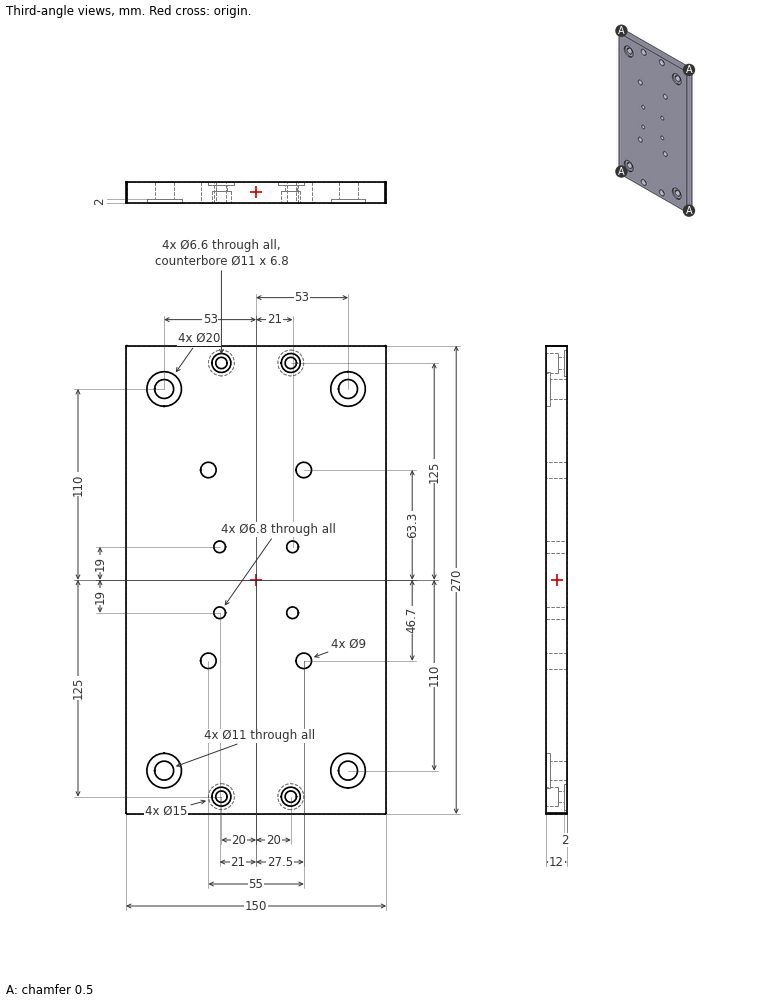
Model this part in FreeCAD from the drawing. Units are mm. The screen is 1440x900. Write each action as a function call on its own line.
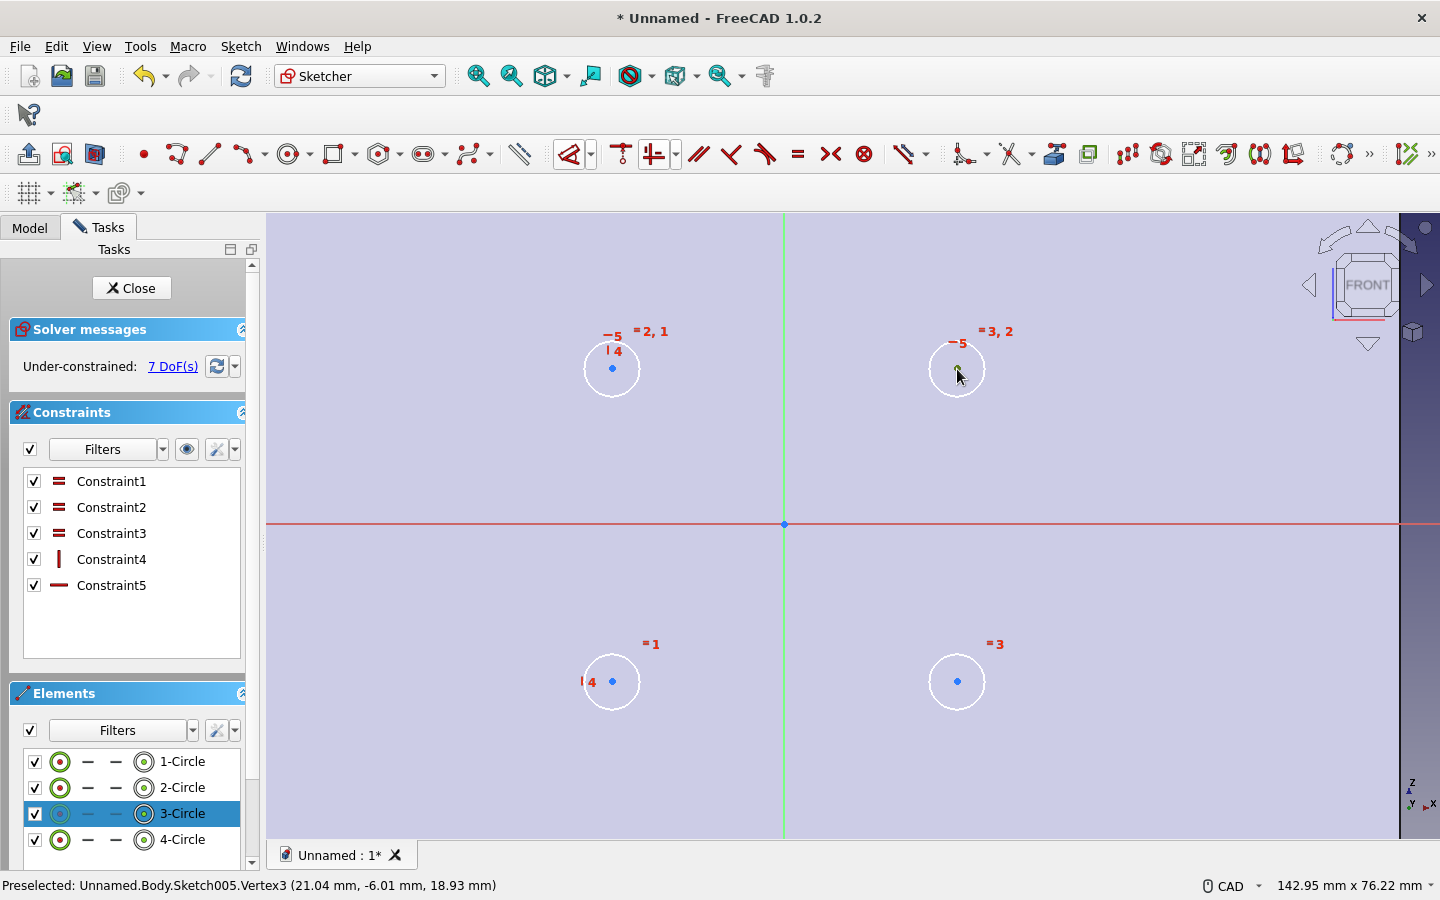
click(957, 682)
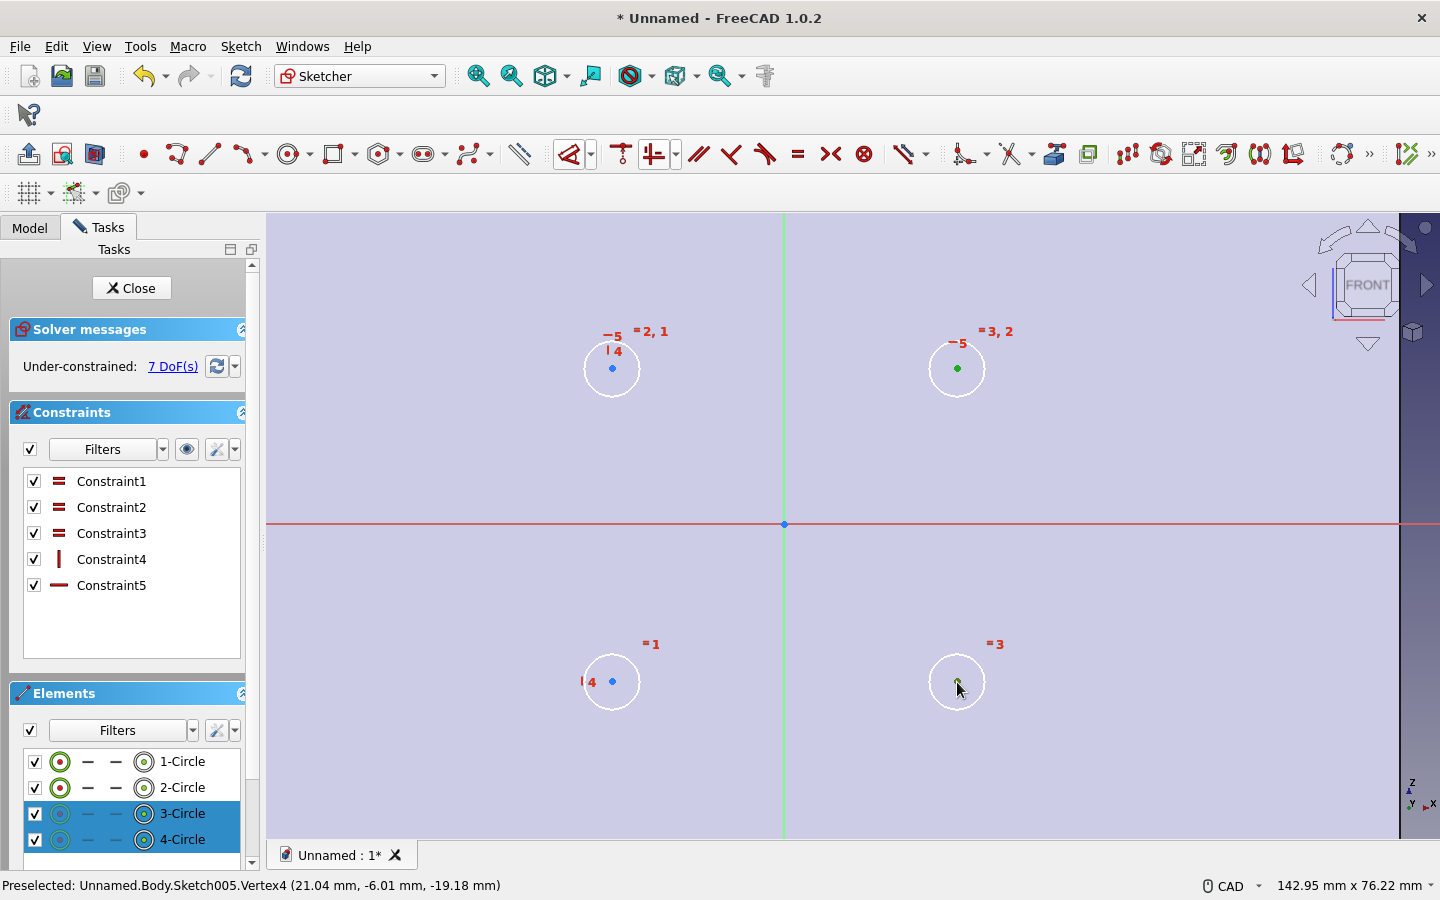
key(v)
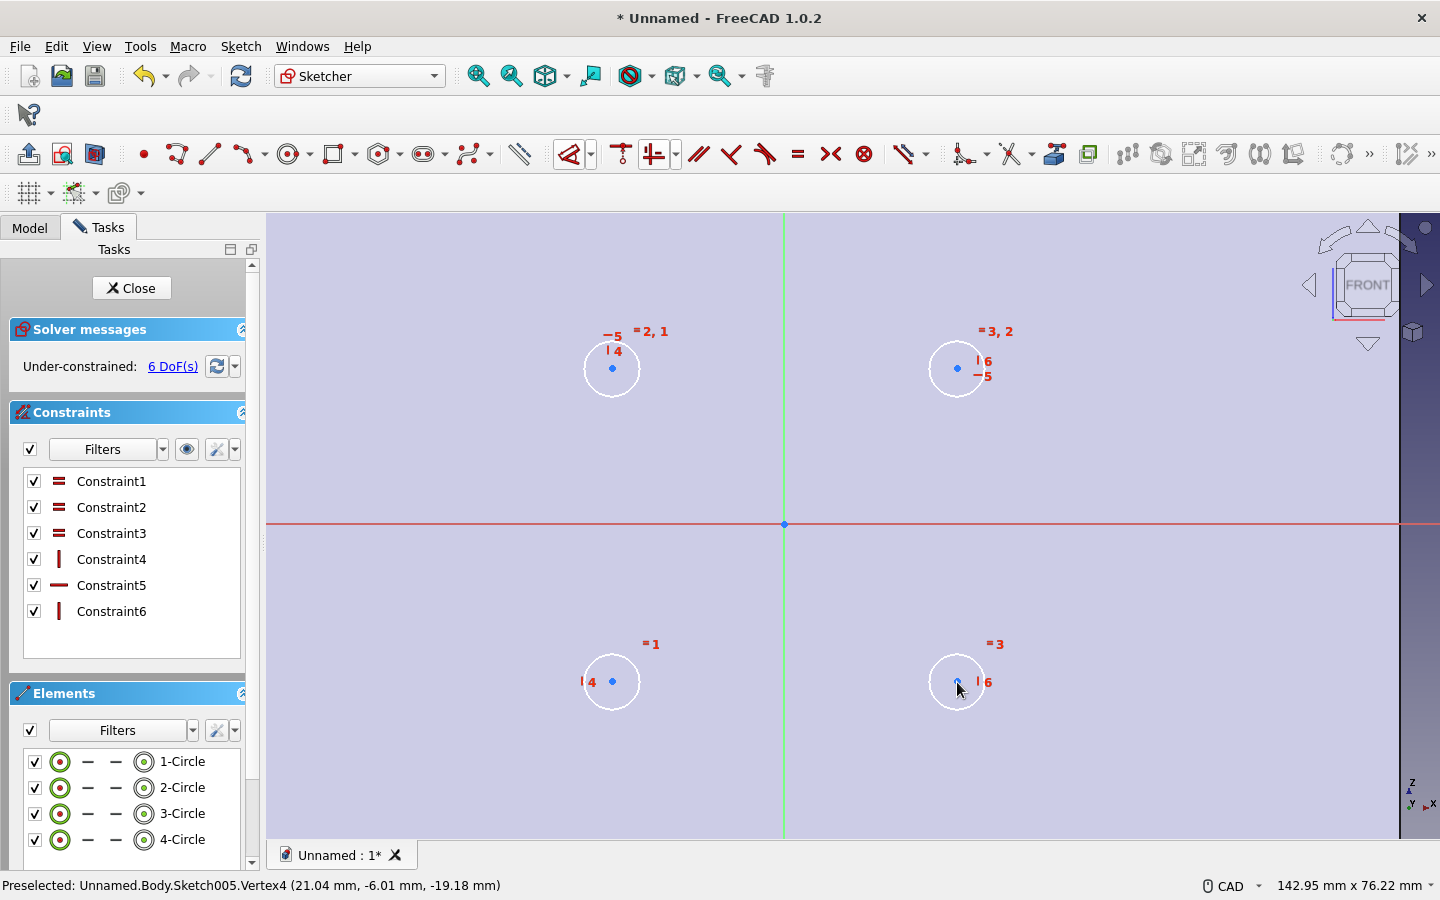
click(612, 682)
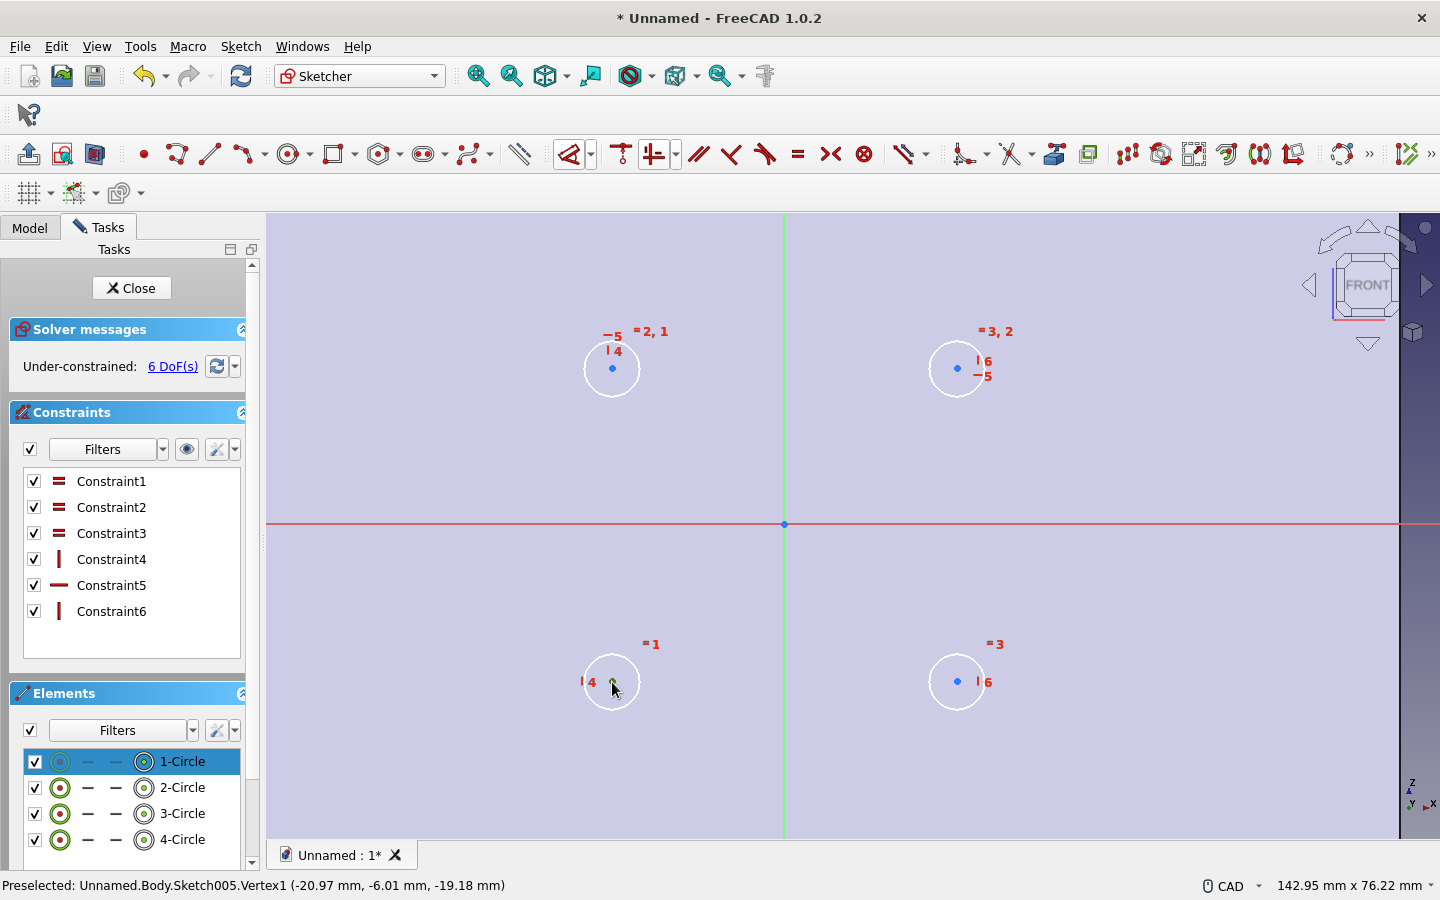
click(957, 682)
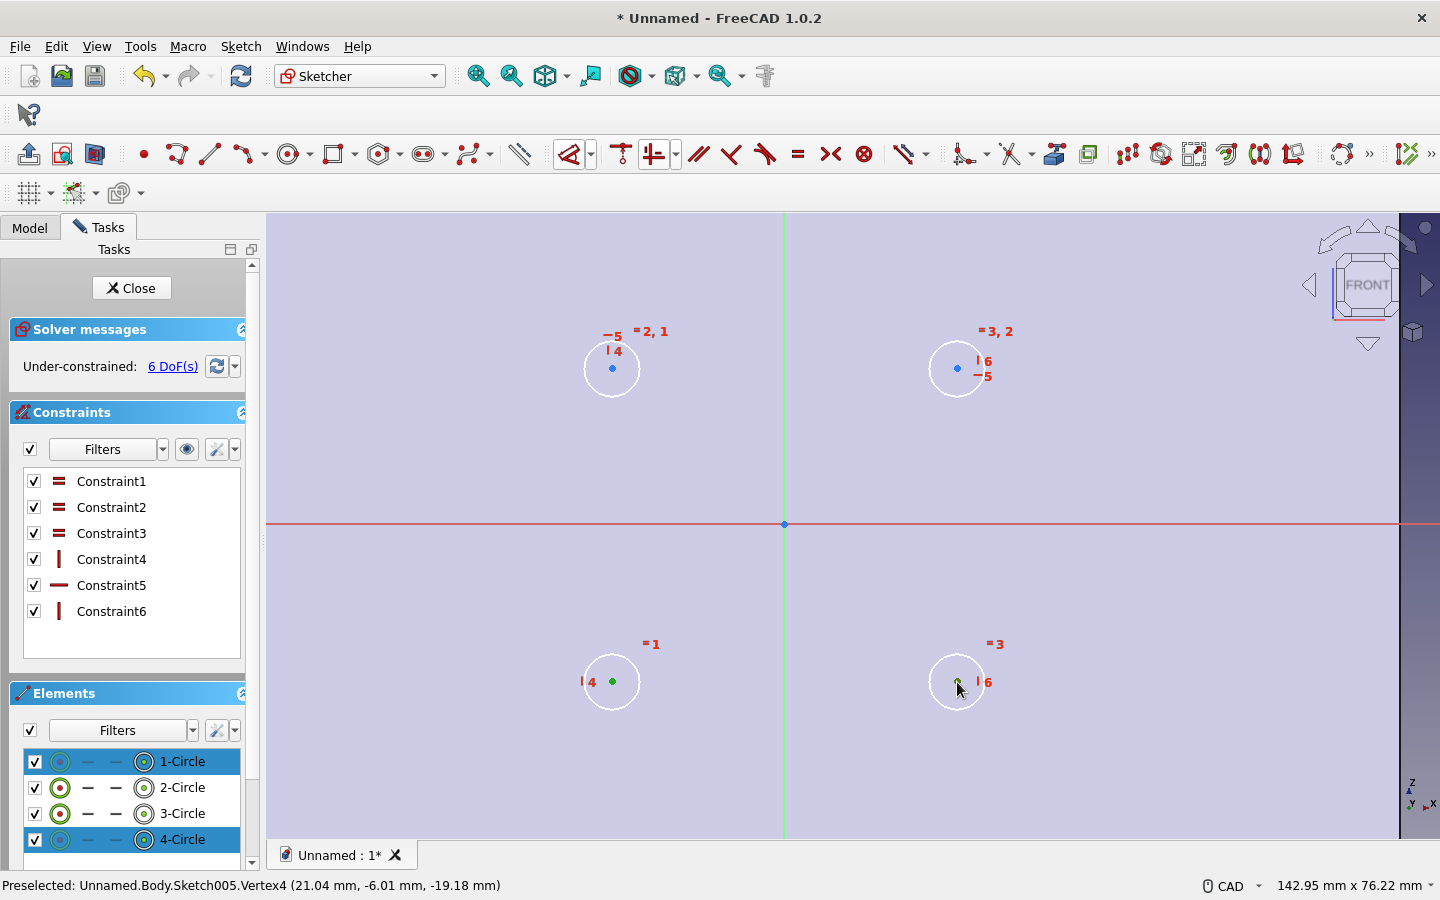
key(h)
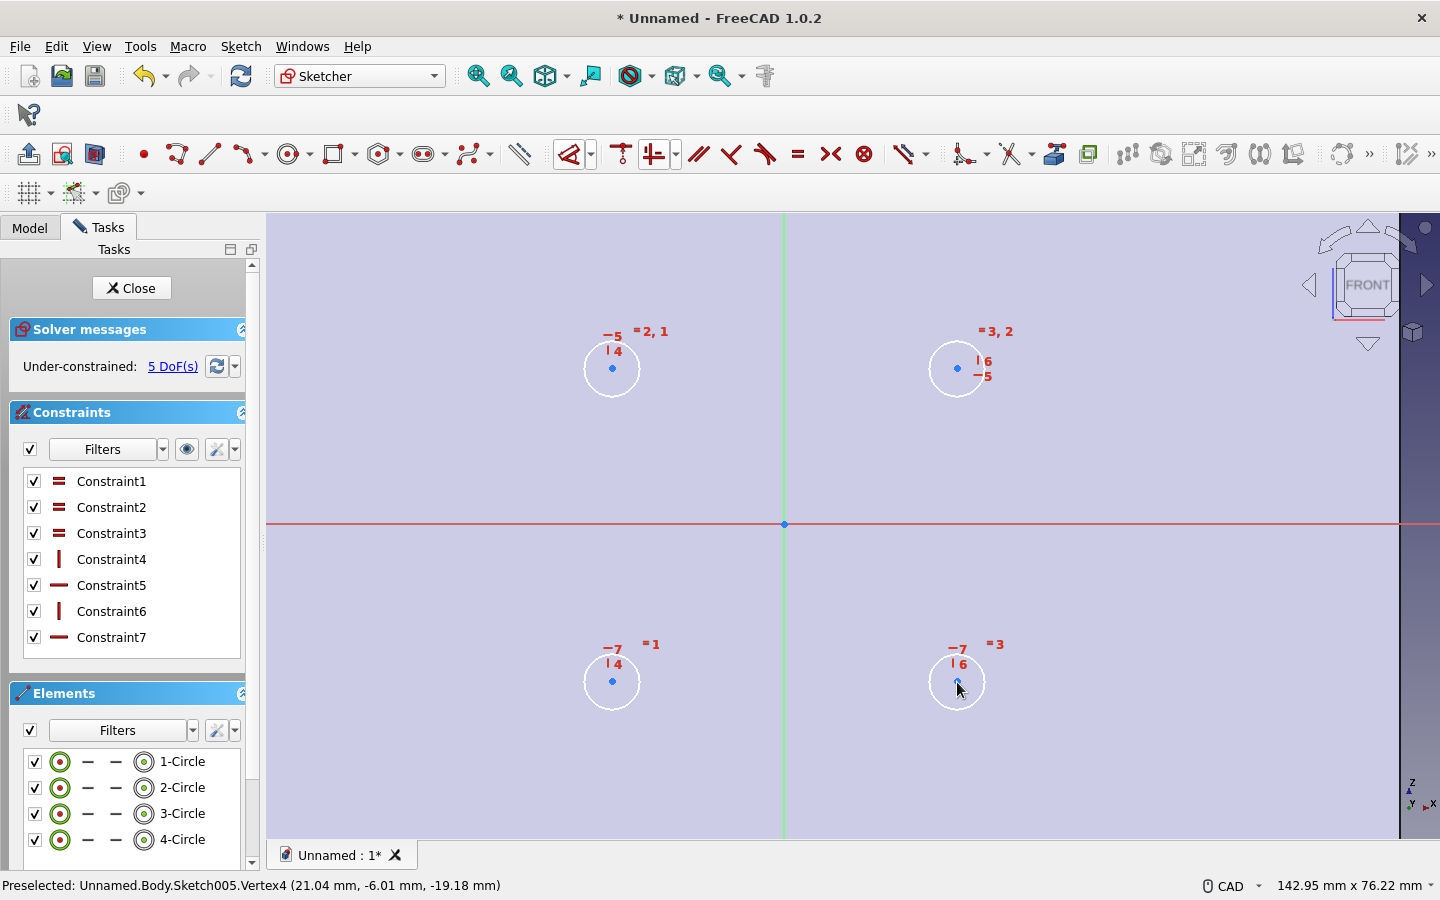
click(631, 662)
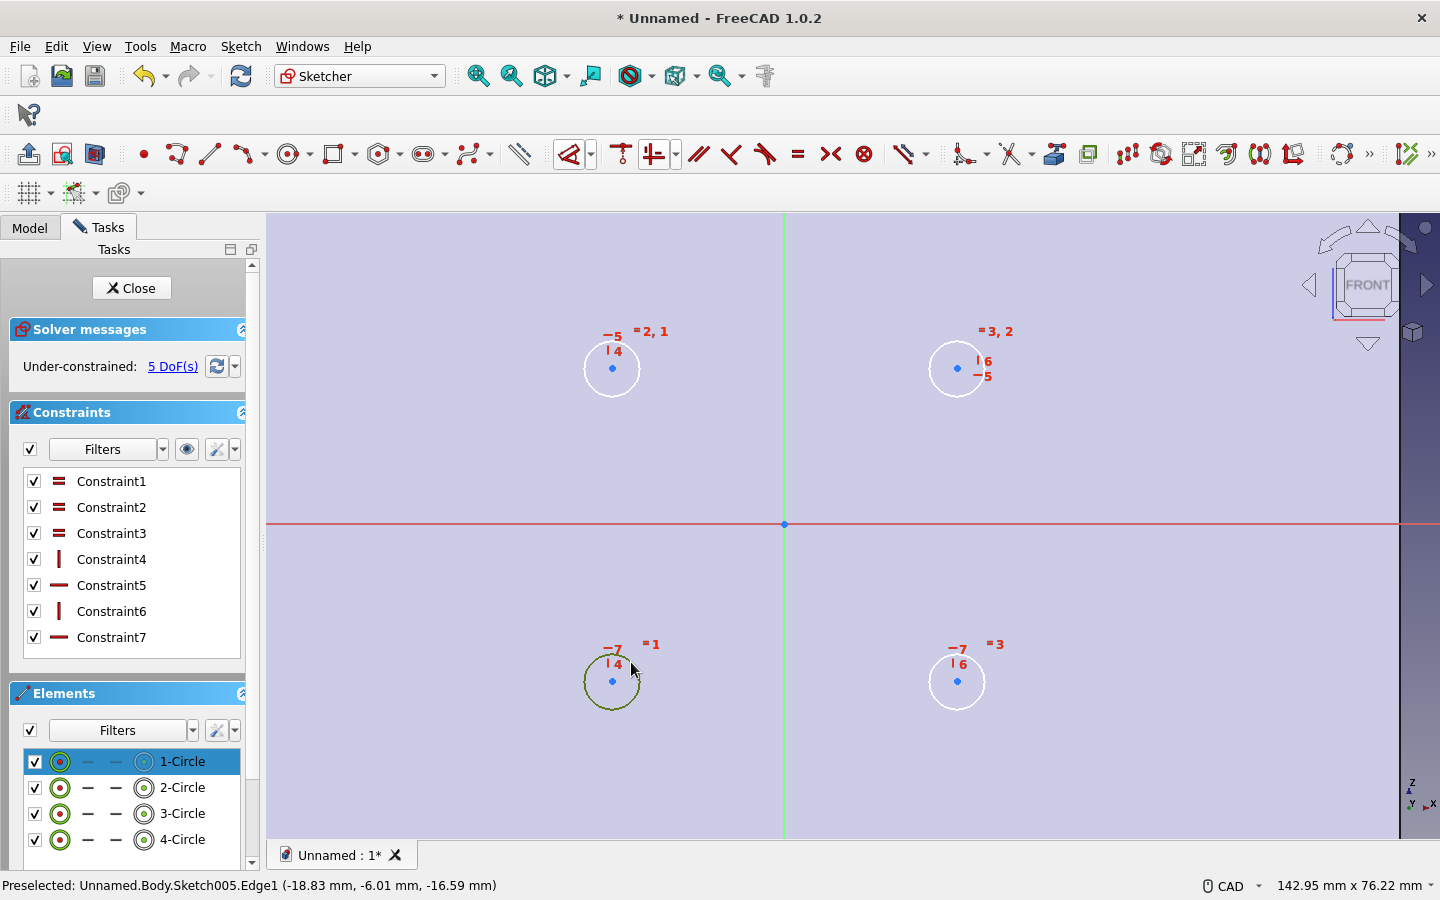
key(k)
key(o)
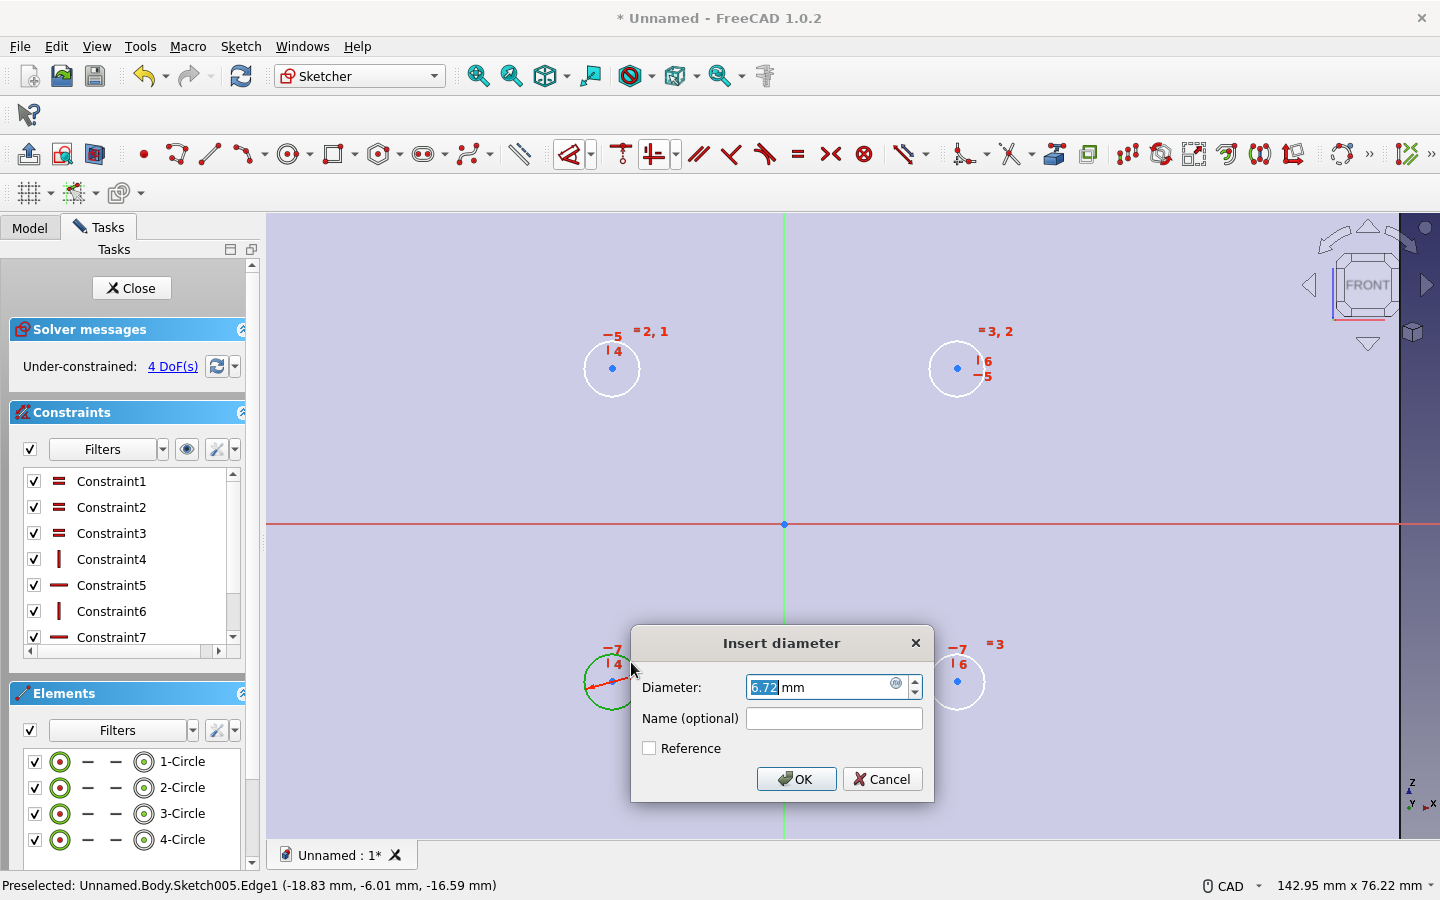
text(6.8)
key(Return)